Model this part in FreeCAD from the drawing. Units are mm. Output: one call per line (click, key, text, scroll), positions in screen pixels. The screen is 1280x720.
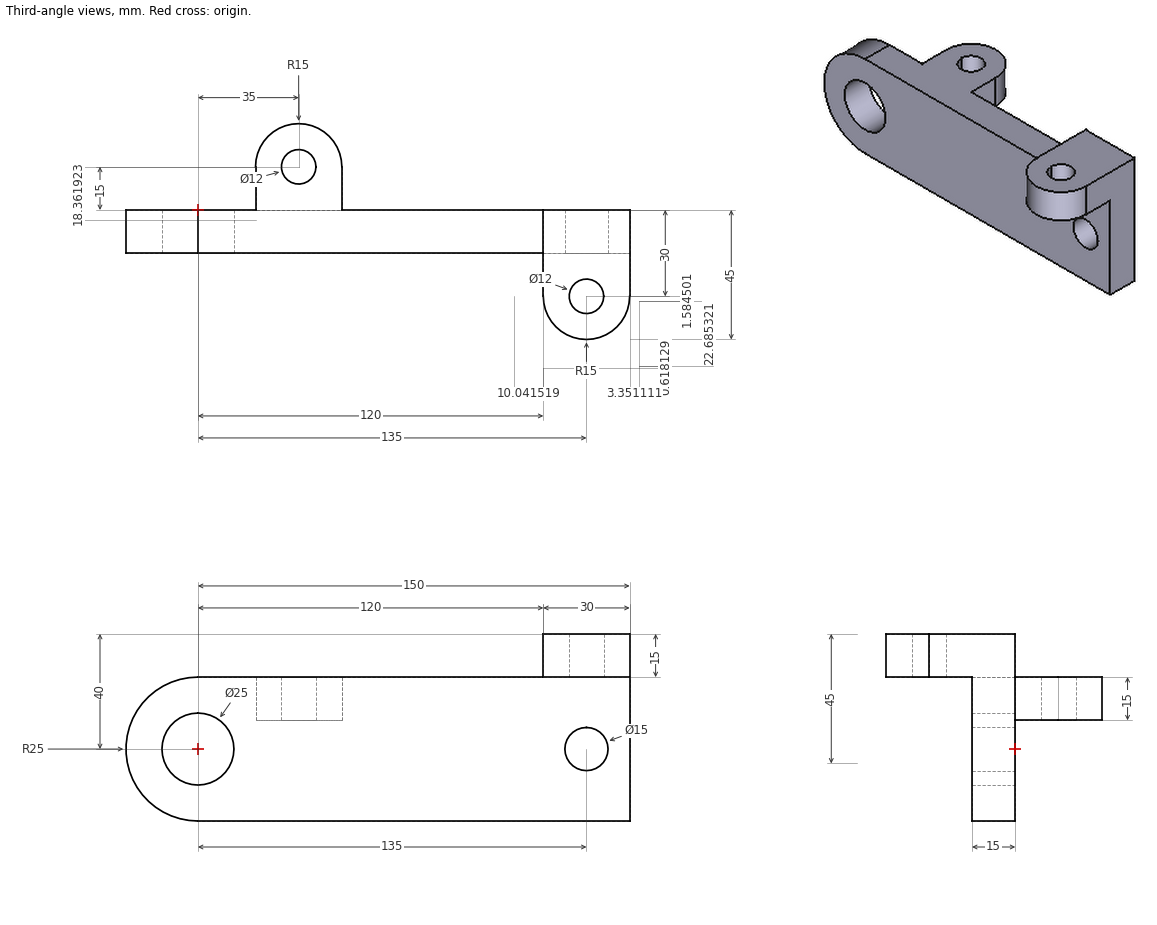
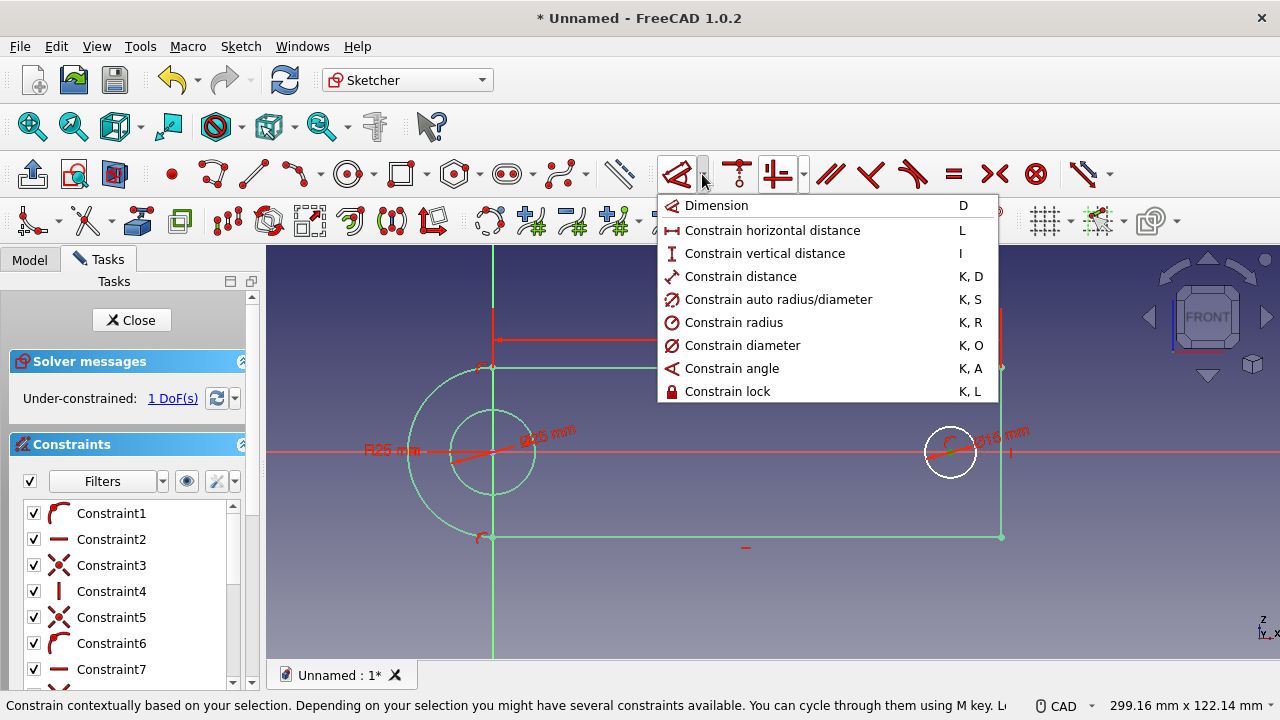
click(828, 230)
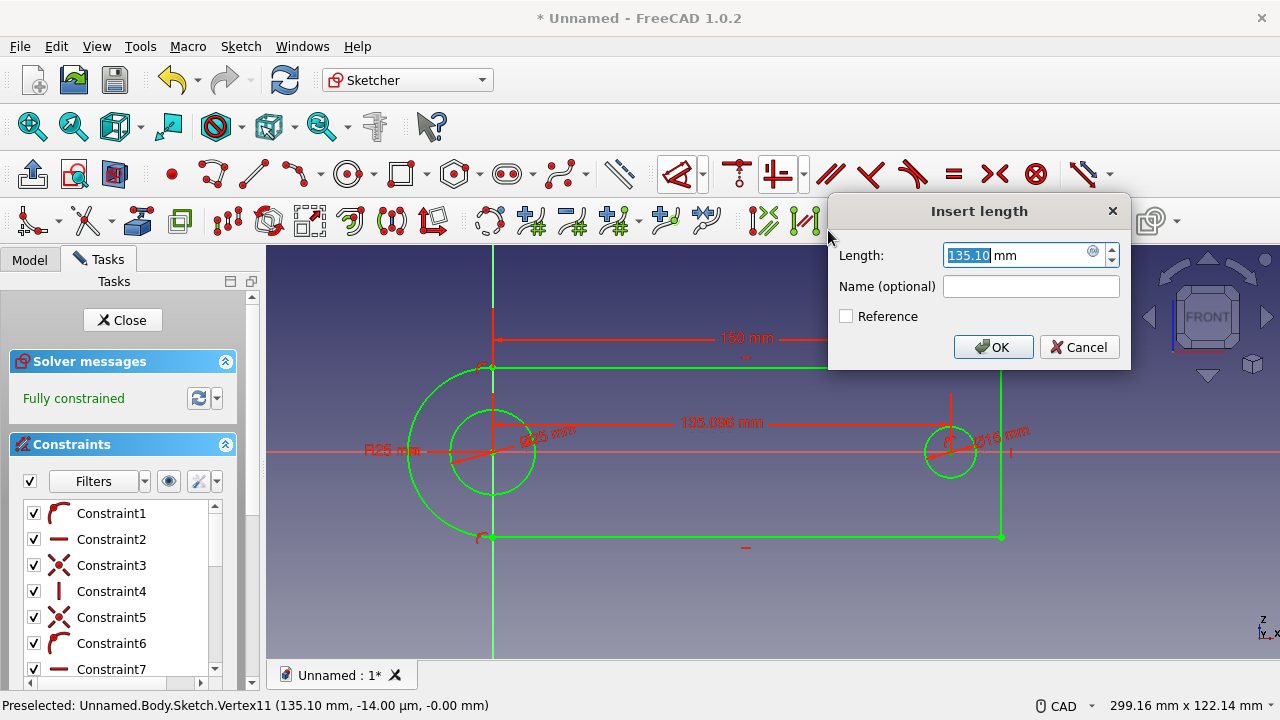
text(135)
key(Return)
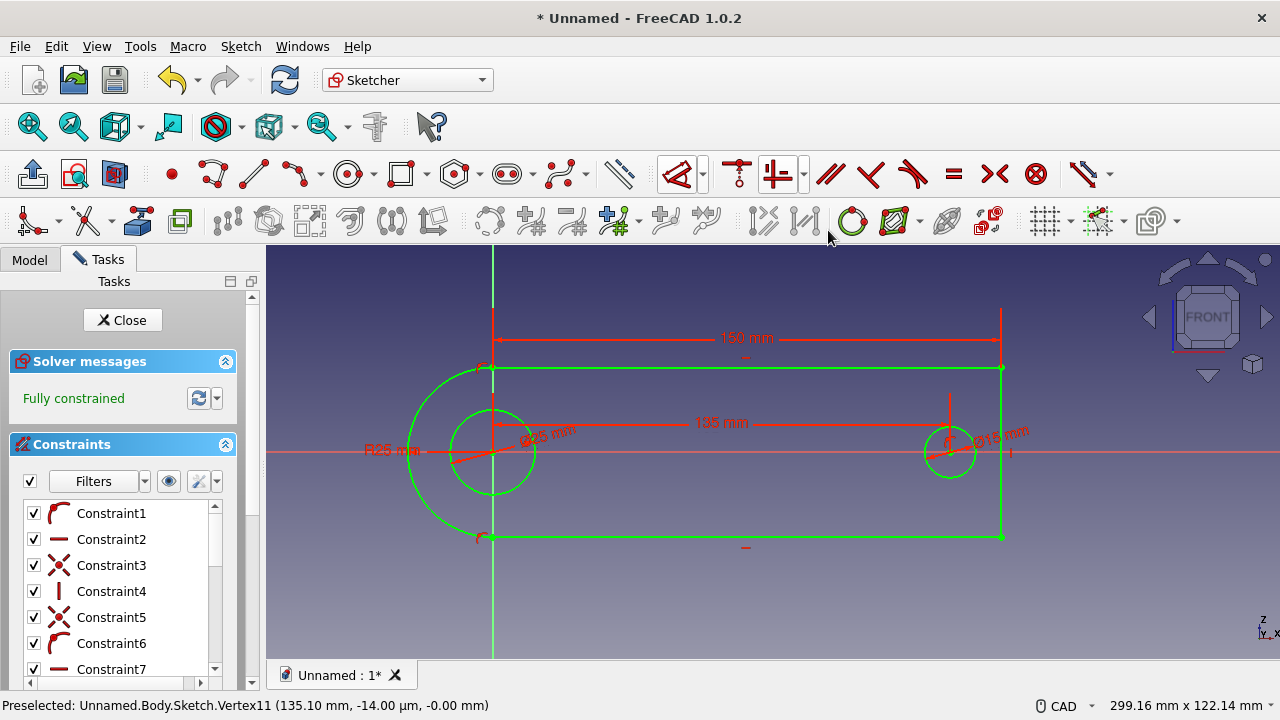
click(123, 320)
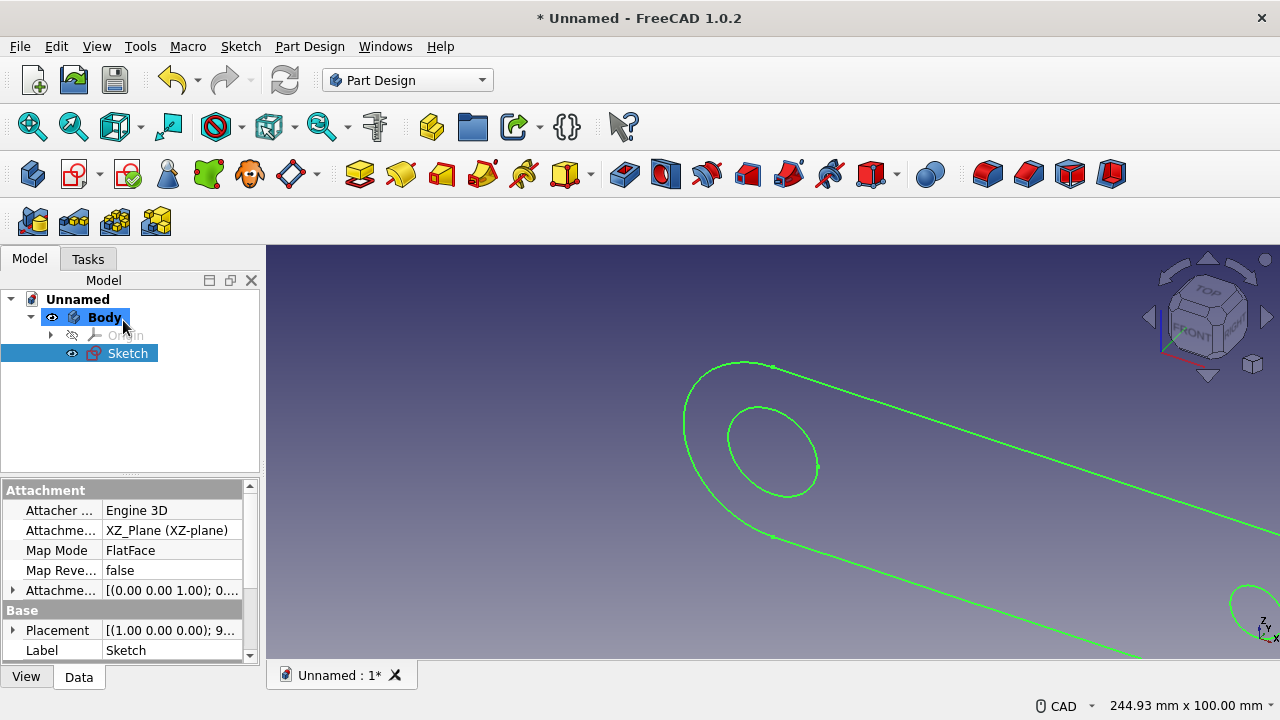
click(360, 174)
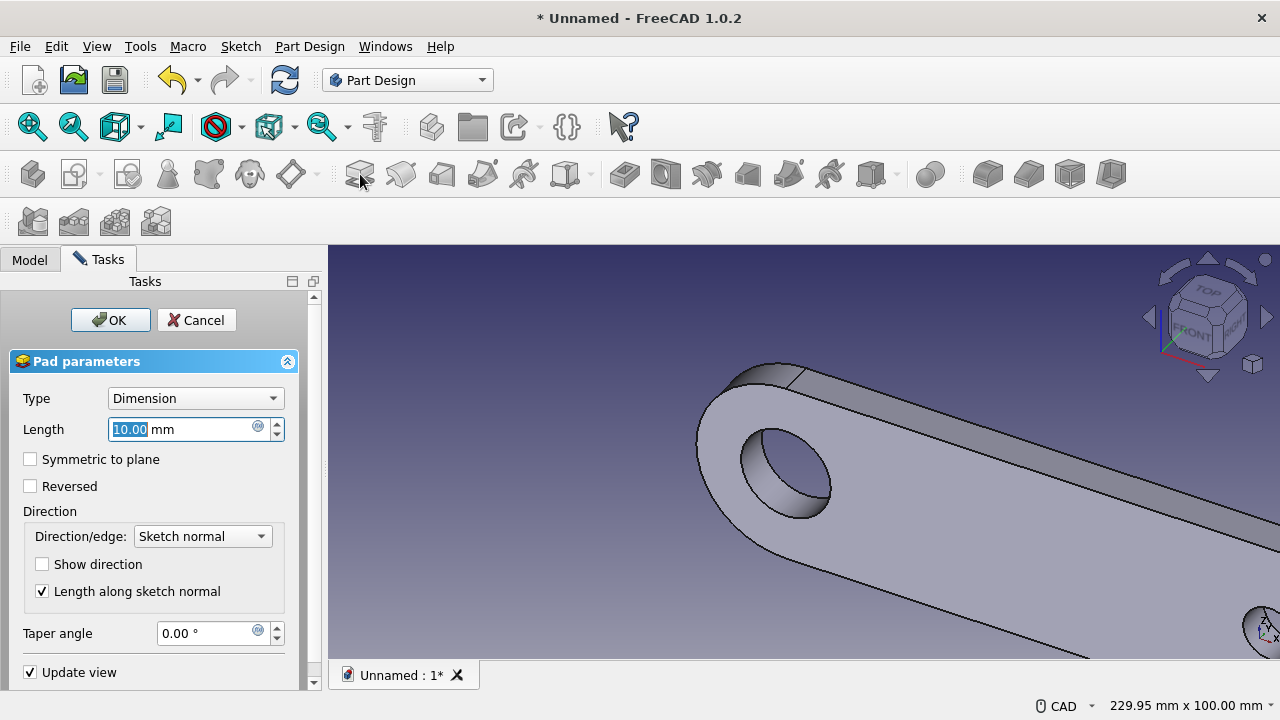
text(15)
key(Tab)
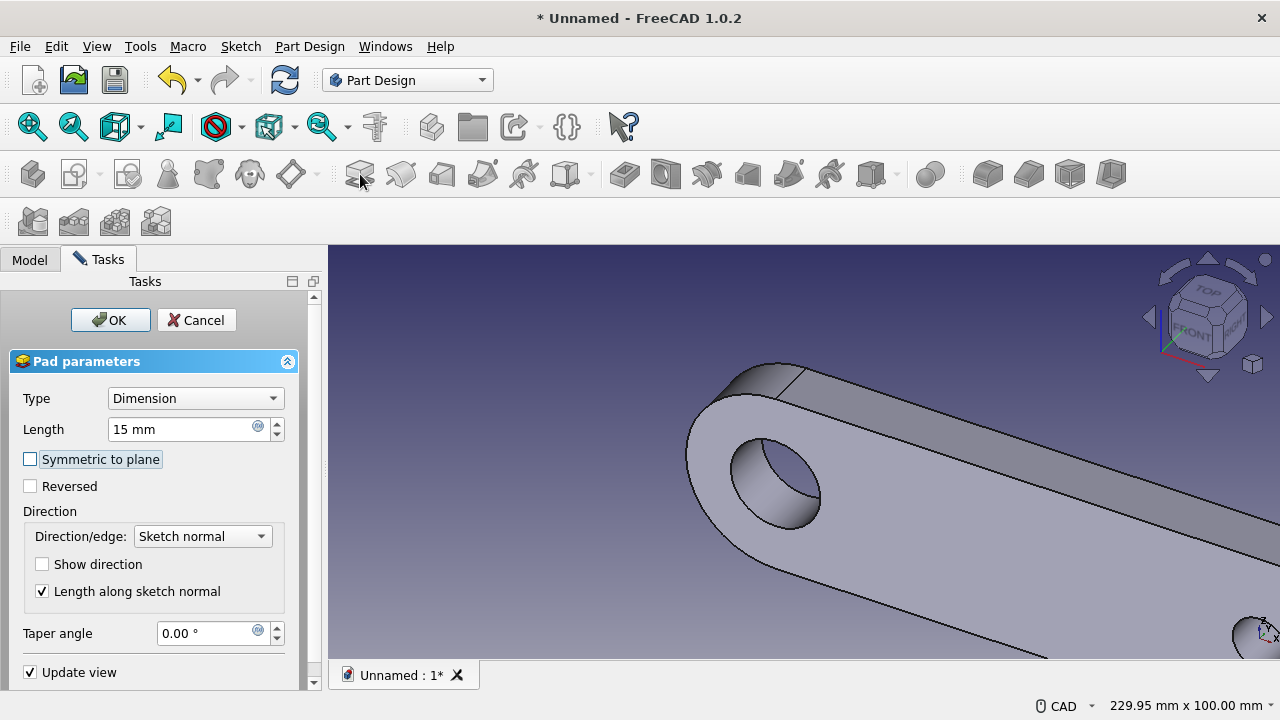
click(111, 320)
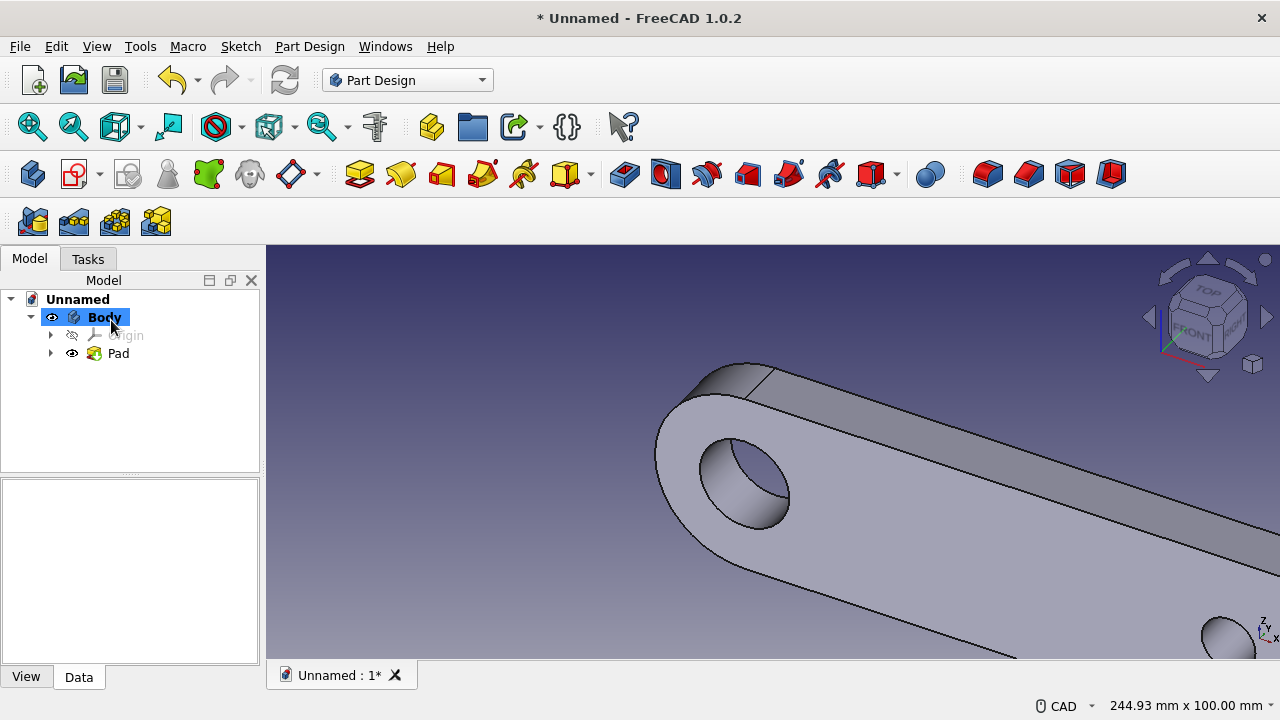
click(33, 128)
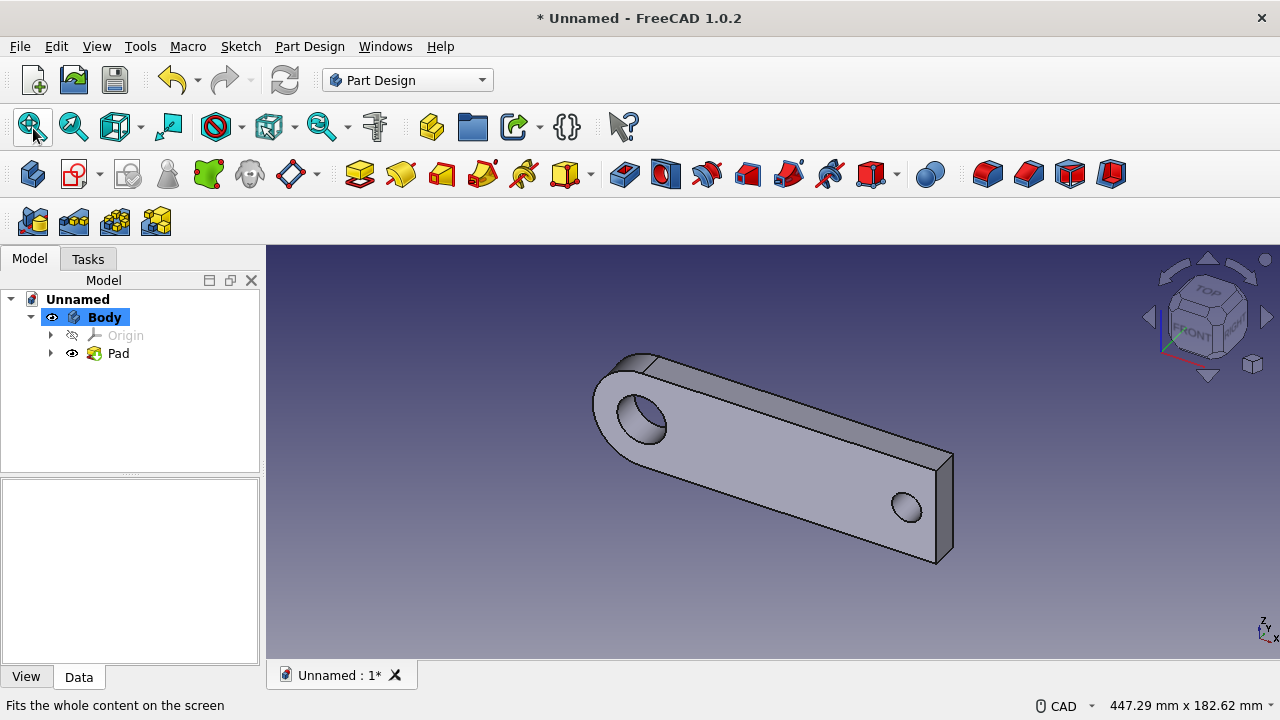
click(74, 174)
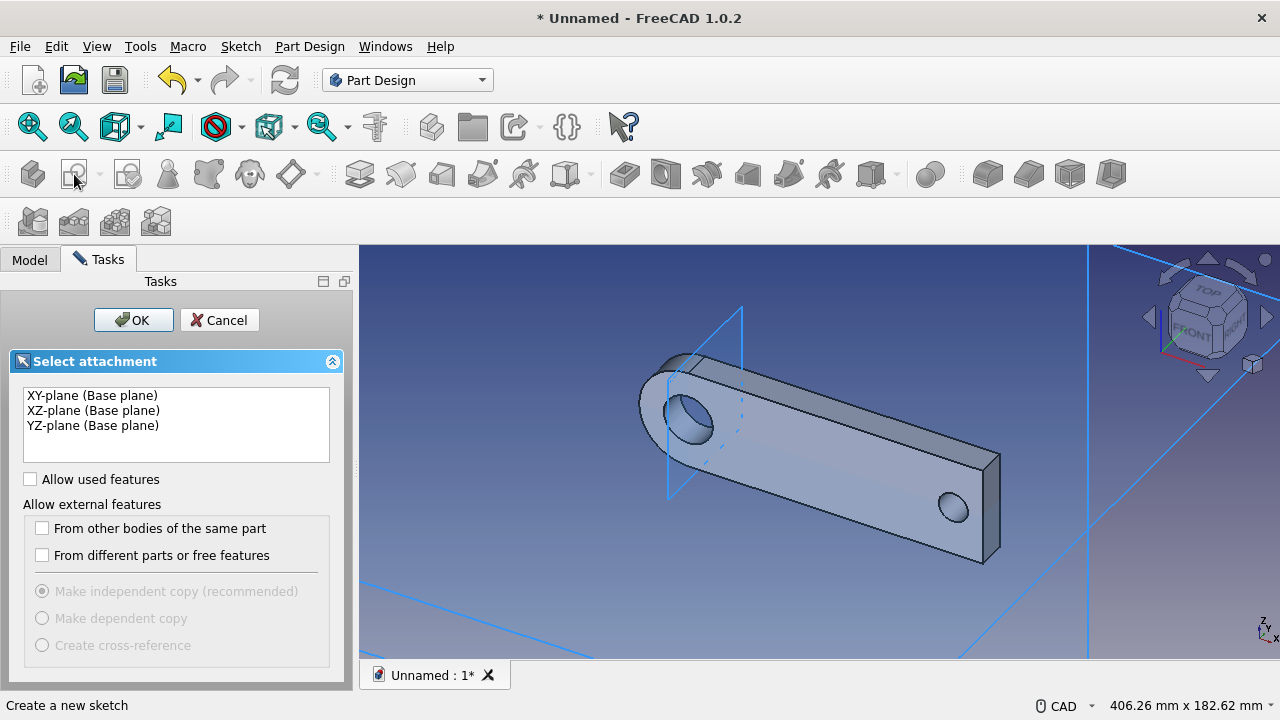
click(84, 410)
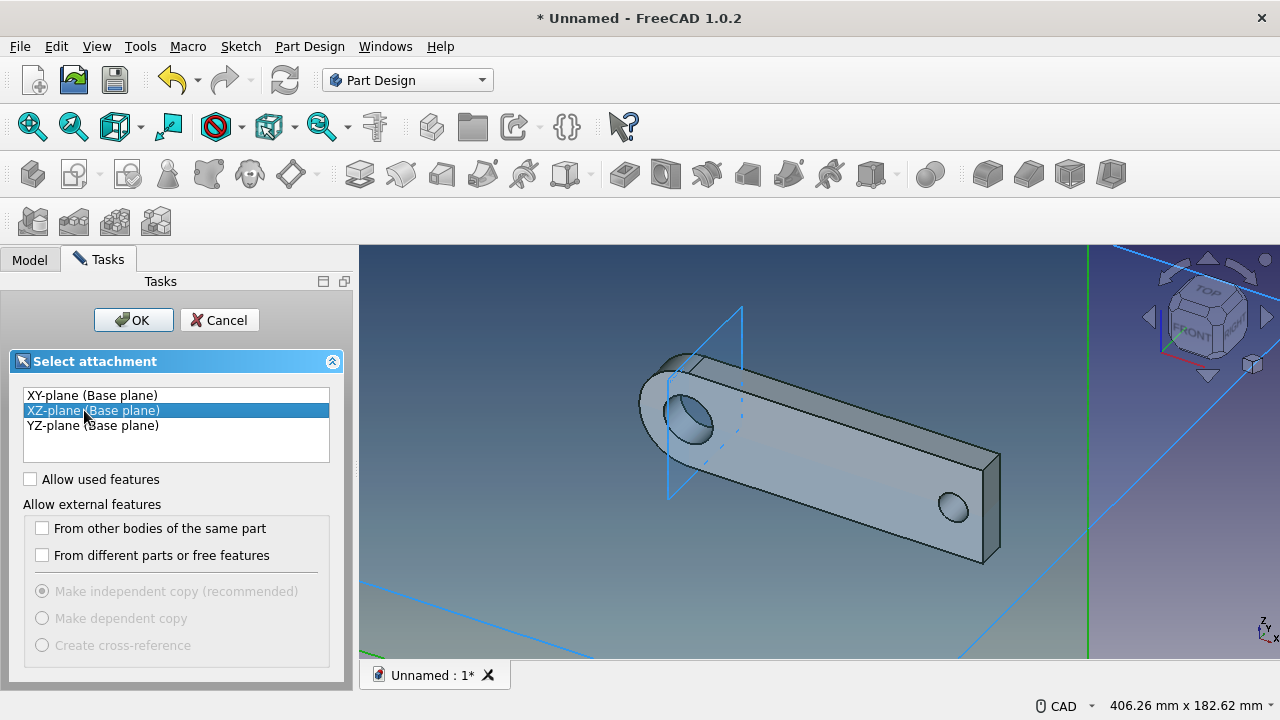
click(134, 320)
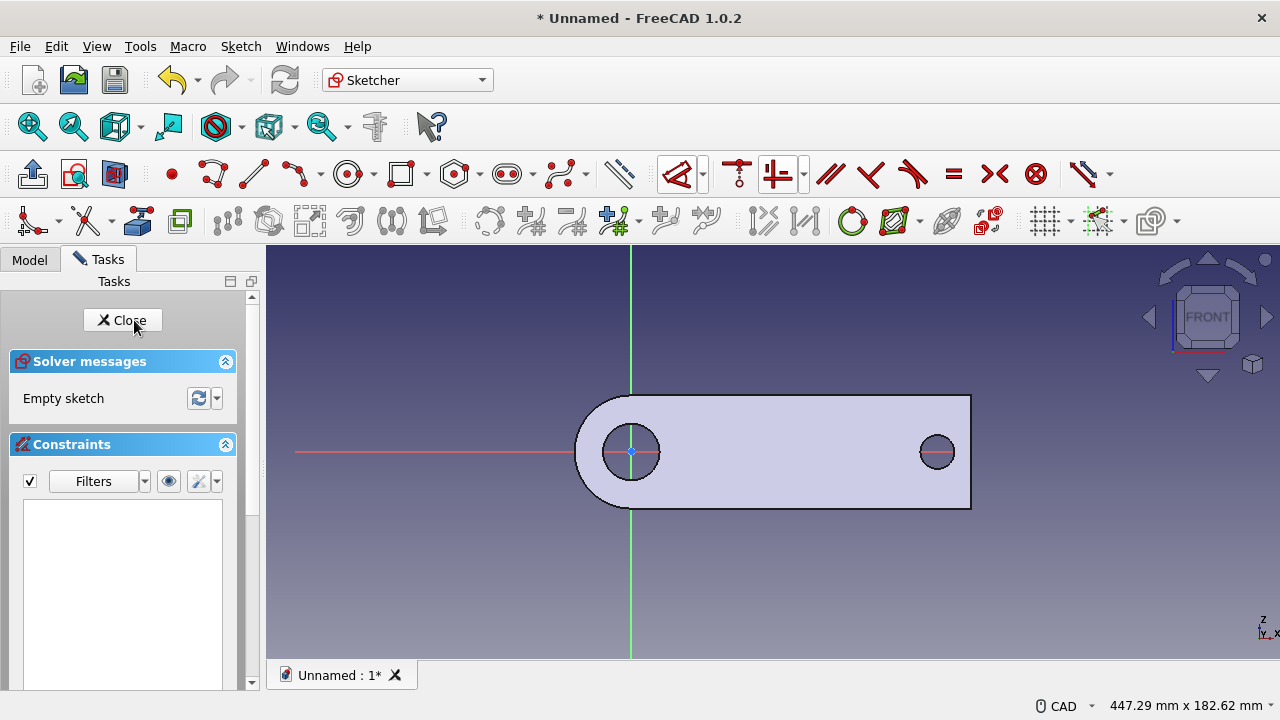
click(115, 174)